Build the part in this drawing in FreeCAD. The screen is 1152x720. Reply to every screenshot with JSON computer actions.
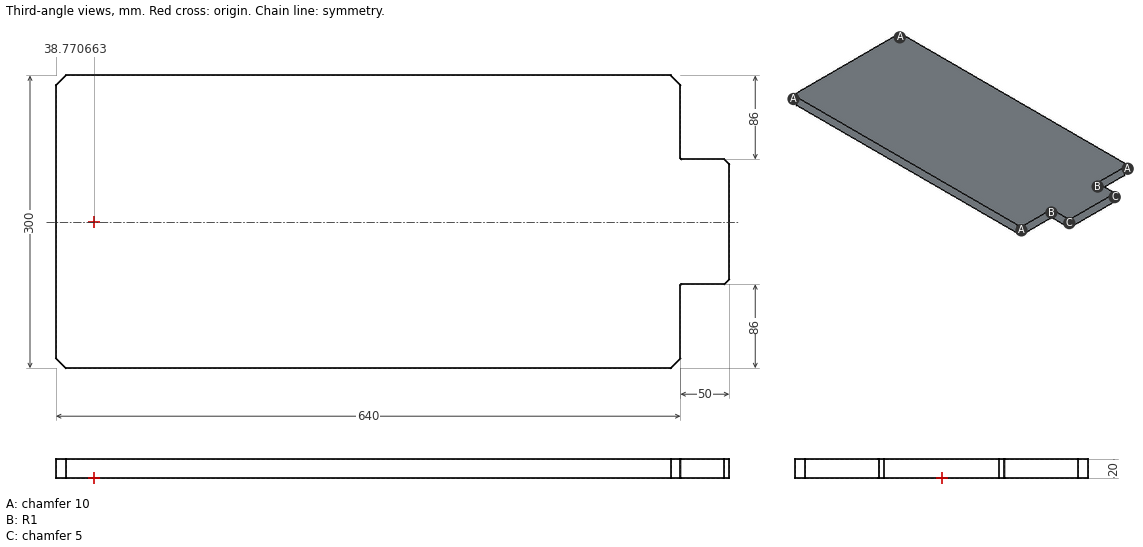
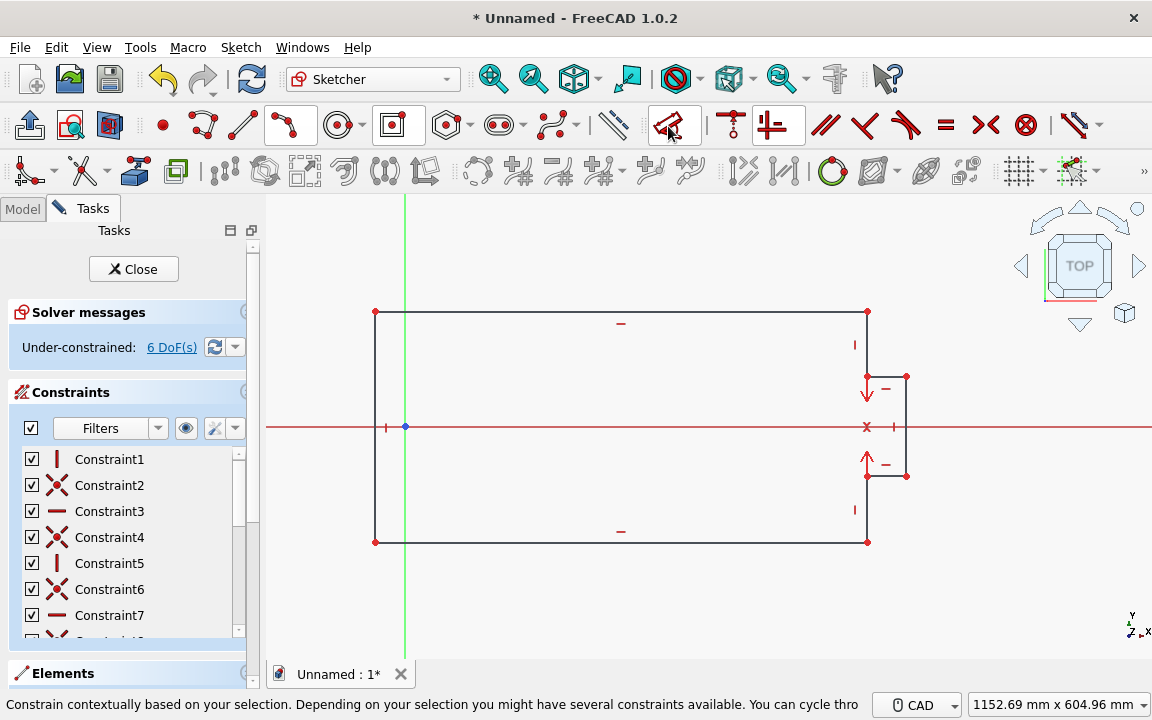
{"action": "left_click", "coordinate": [867, 523]}
{"action": "left_click", "coordinate": [901, 510]}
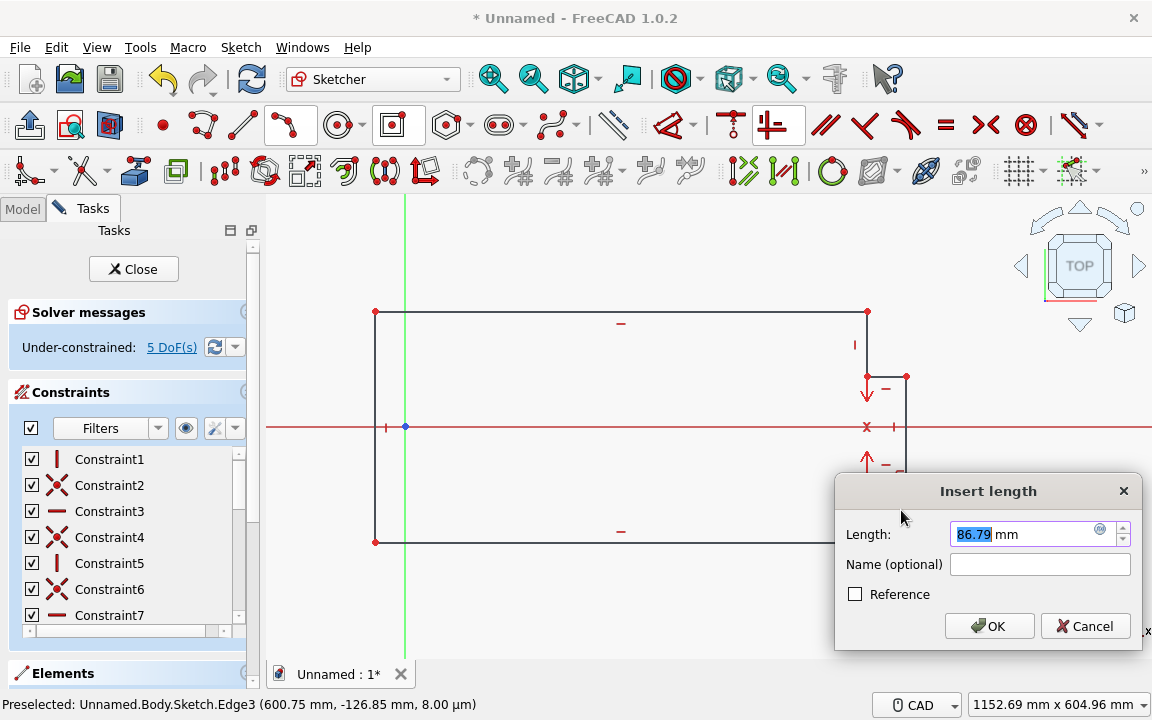
{"action": "type", "text": "86"}
{"action": "key", "text": "Return"}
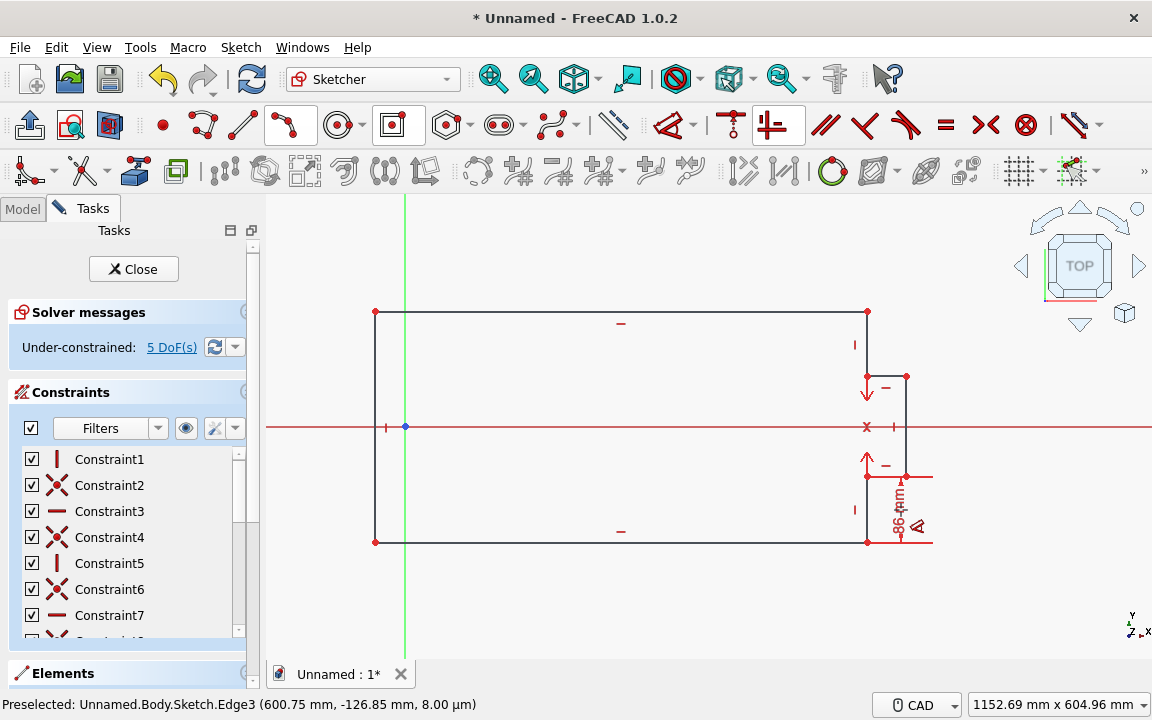
{"action": "left_click", "coordinate": [879, 477]}
{"action": "left_click", "coordinate": [886, 443]}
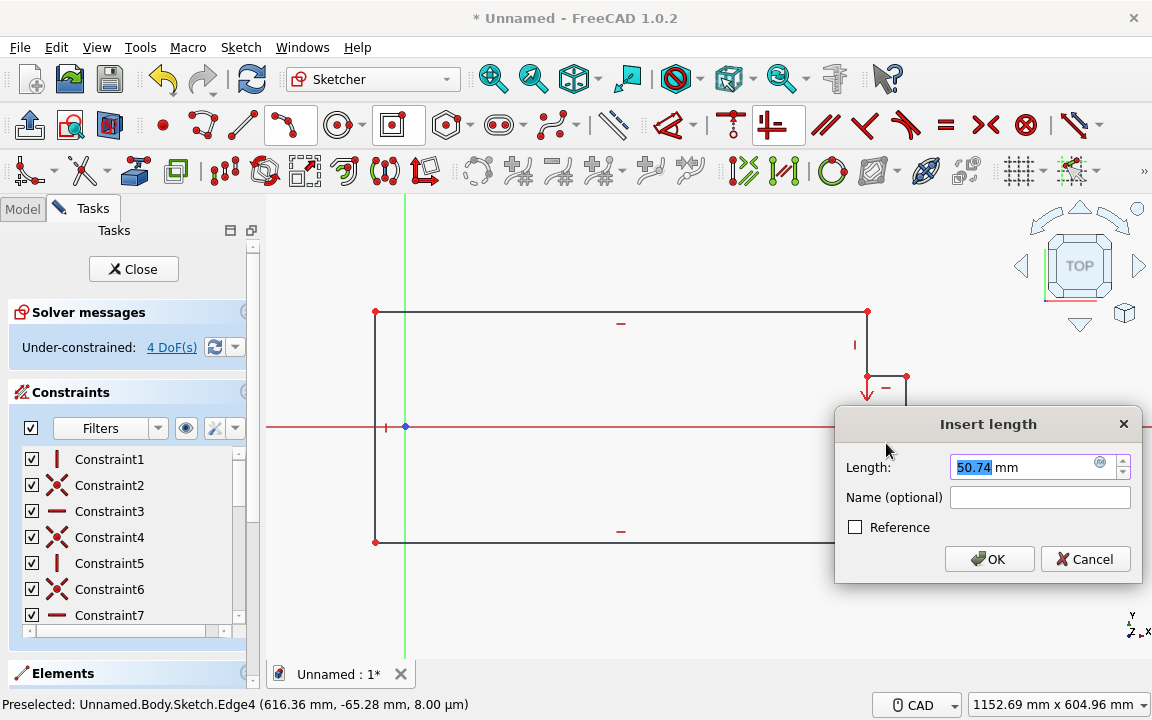
{"action": "type", "text": "50"}
{"action": "key", "text": "Return"}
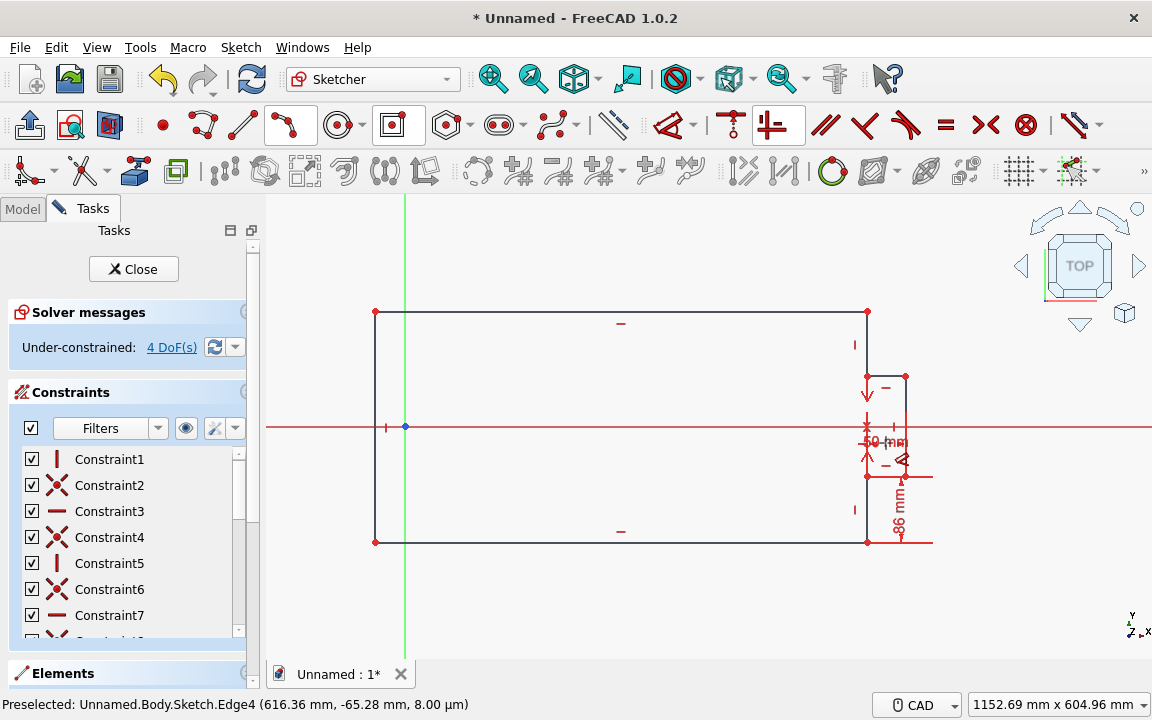
{"action": "left_click", "coordinate": [867, 357]}
{"action": "left_click", "coordinate": [901, 344]}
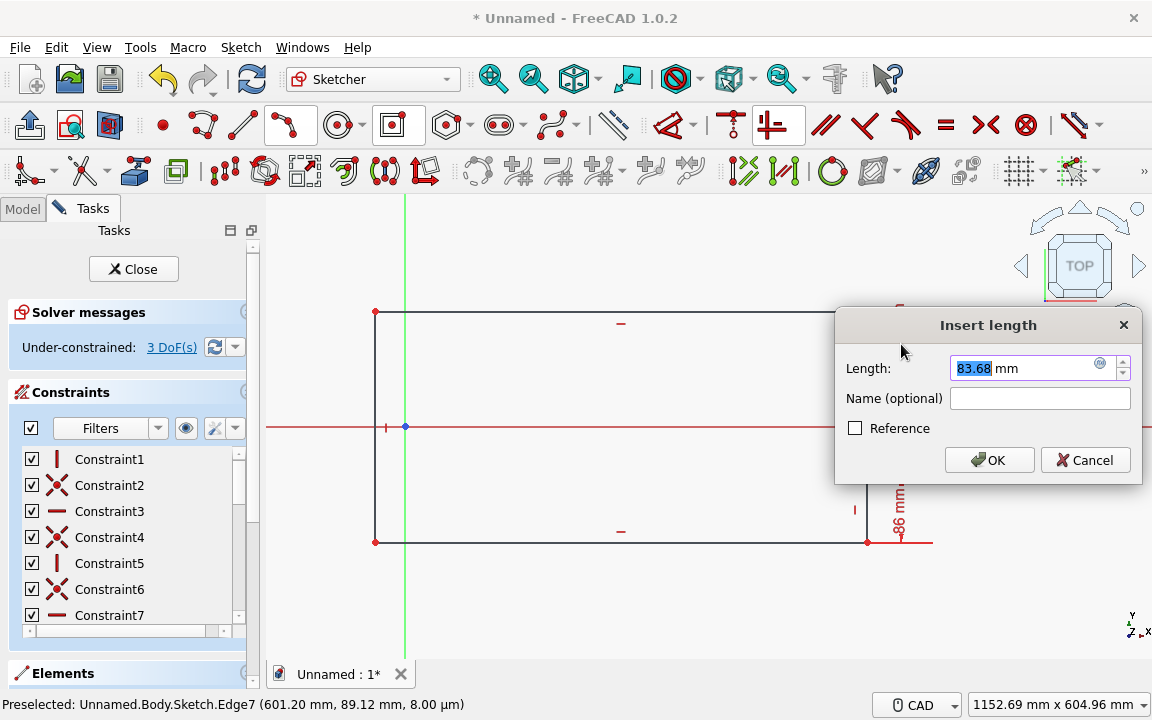
{"action": "type", "text": "86"}
{"action": "key", "text": "Return"}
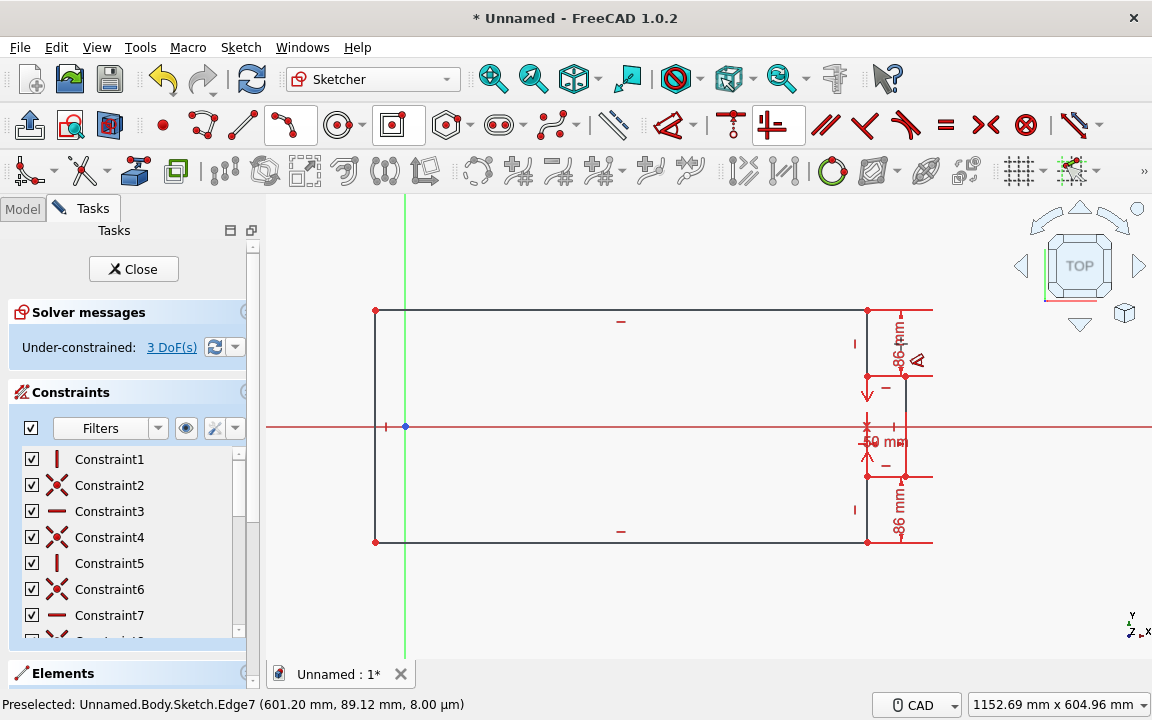
{"action": "left_click", "coordinate": [375, 380]}
{"action": "left_click", "coordinate": [341, 373]}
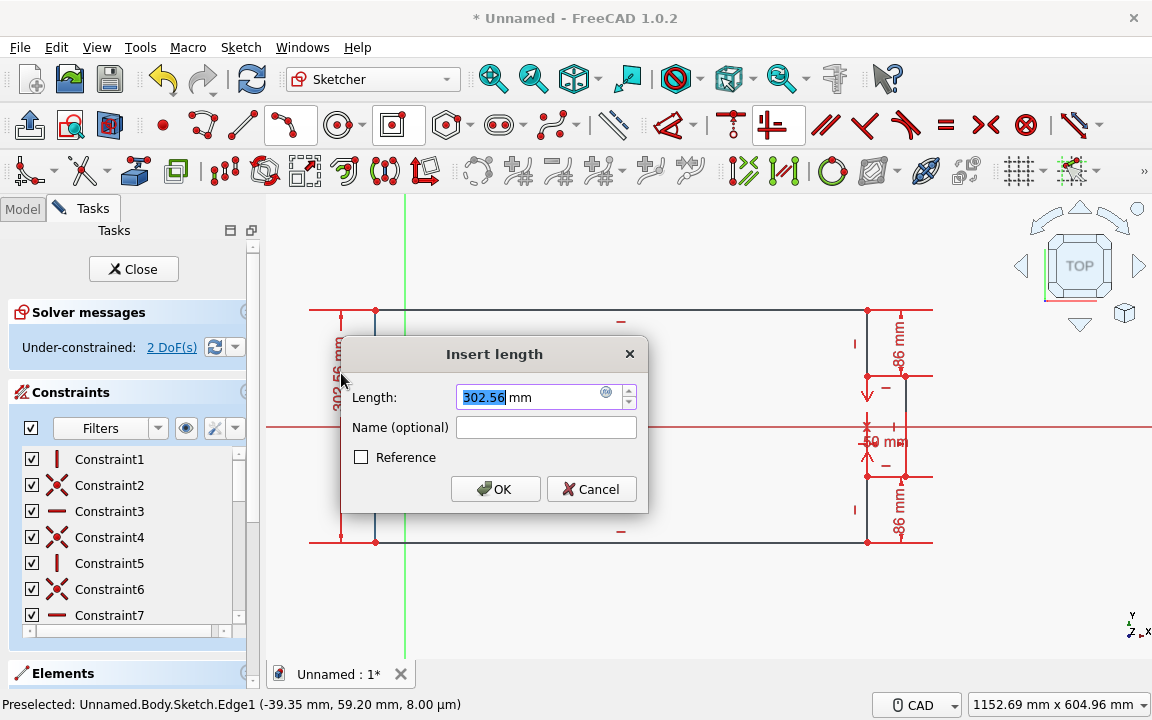
{"action": "type", "text": "300"}
{"action": "key", "text": "Return"}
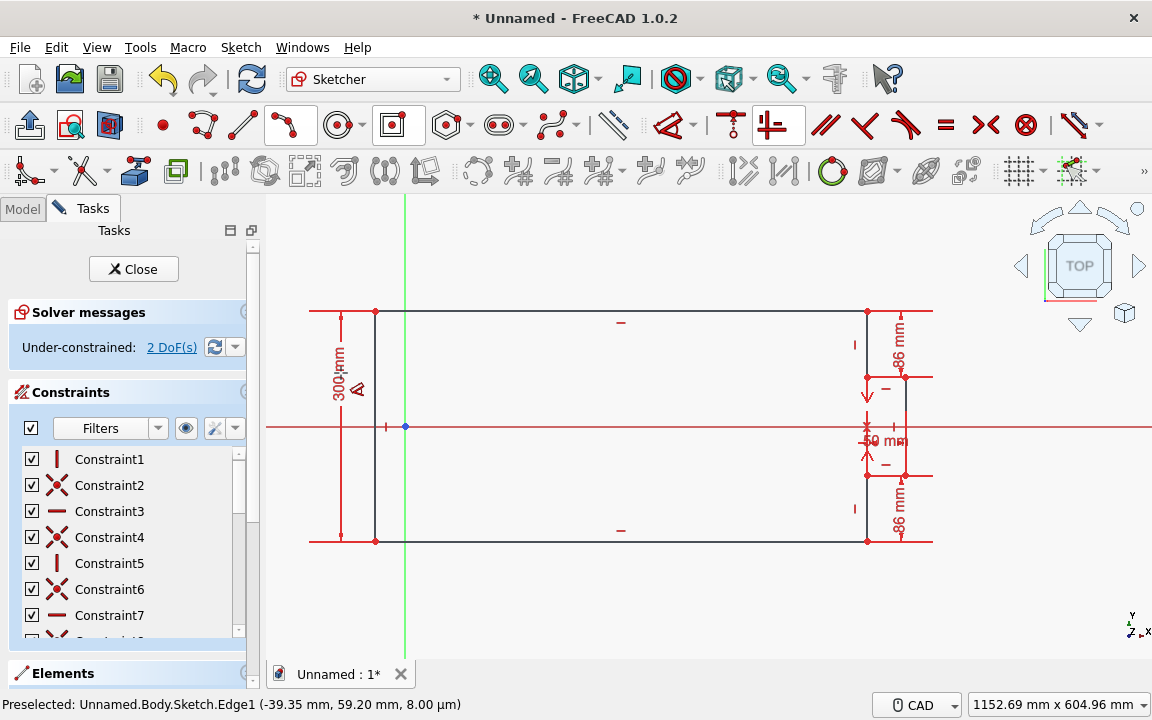
{"action": "left_click", "coordinate": [523, 542]}
{"action": "left_click", "coordinate": [621, 576]}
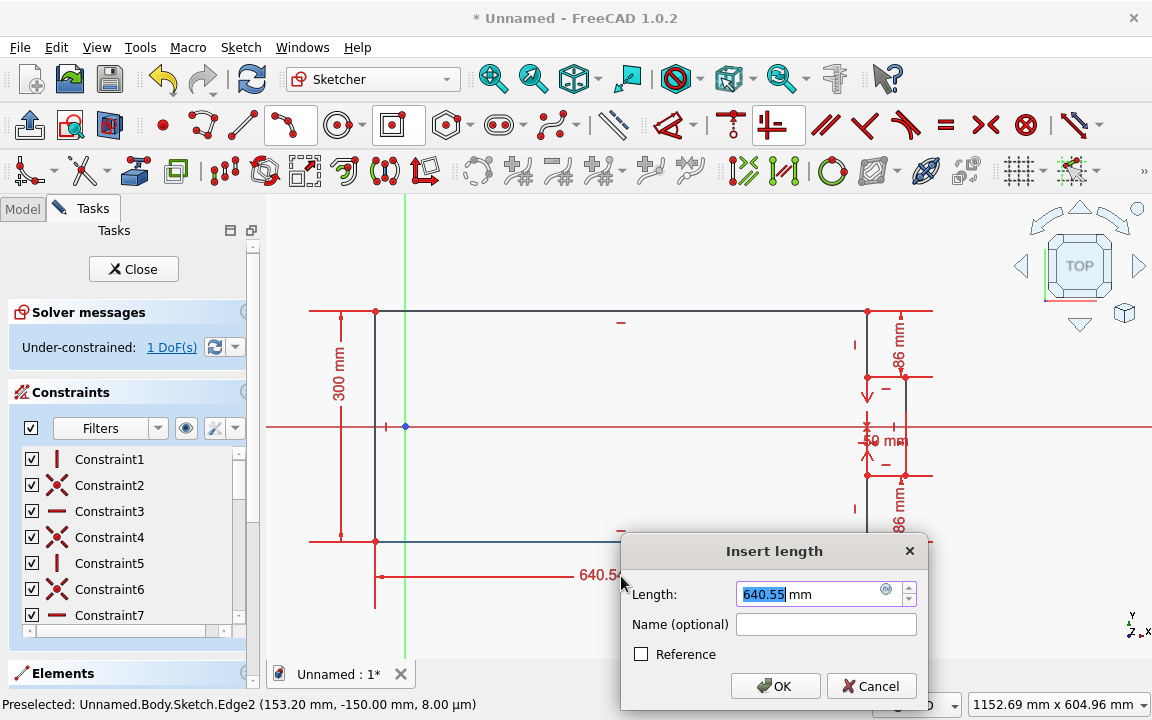
{"action": "type", "text": "640"}
{"action": "key", "text": "Return"}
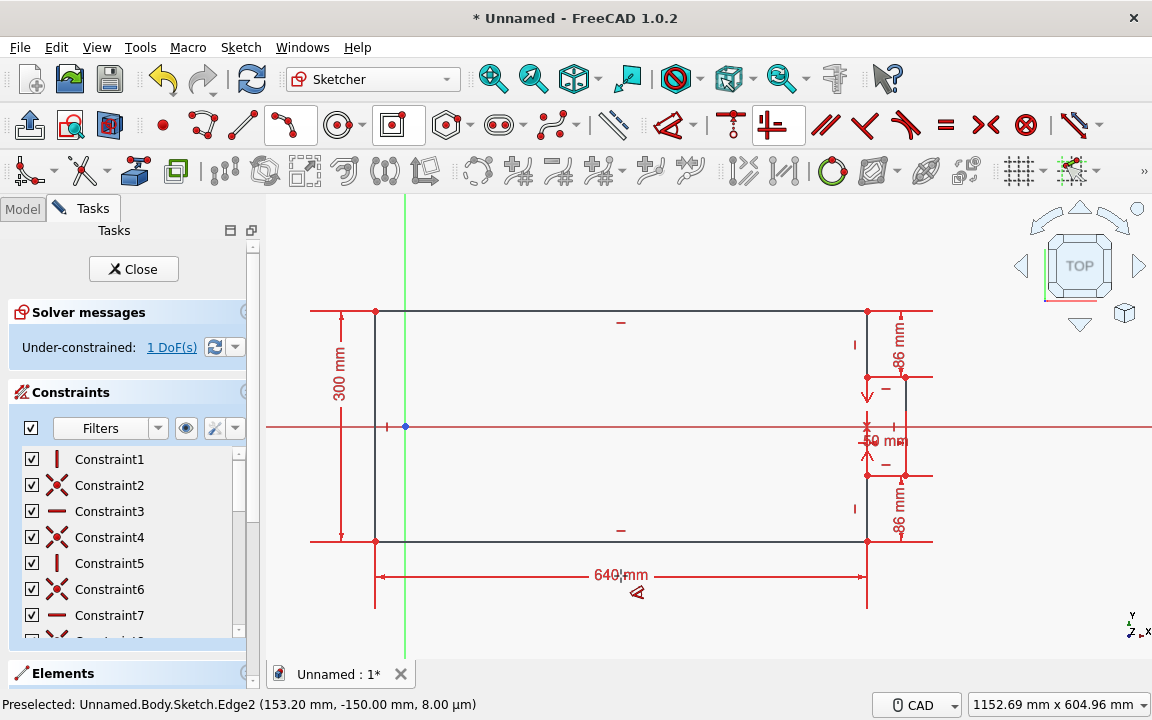
{"action": "scroll", "coordinate": [375, 311], "scroll_direction": "up", "scroll_amount": 2}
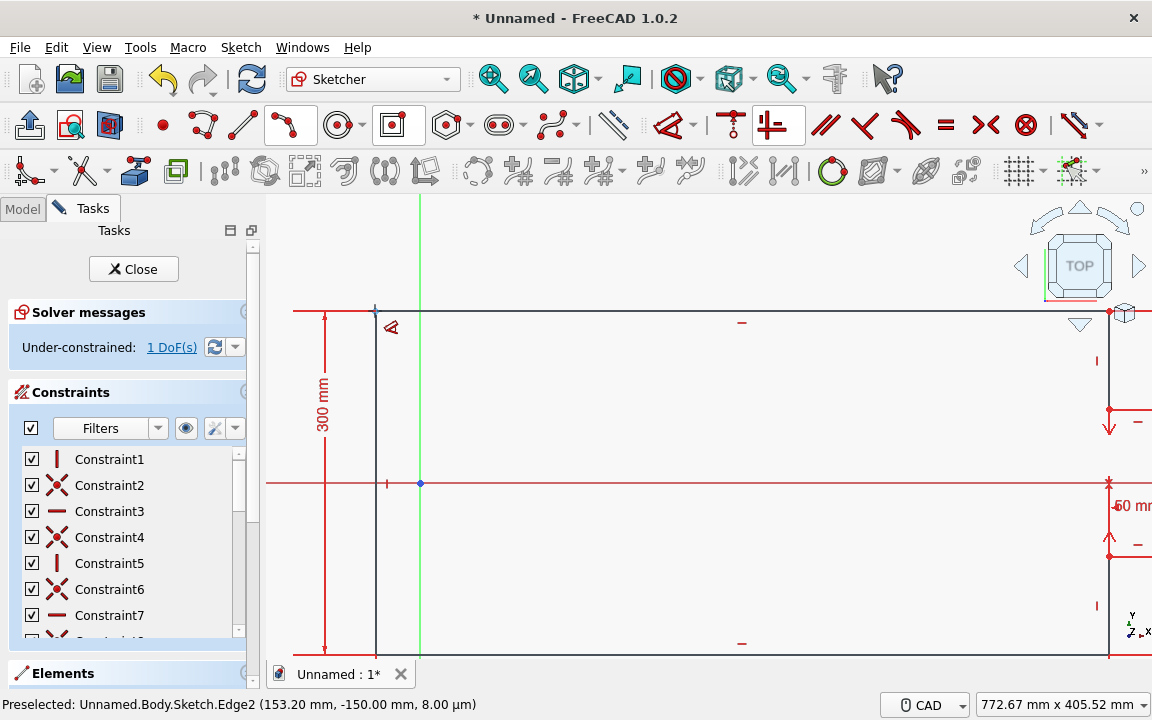
{"action": "left_click", "coordinate": [376, 311]}
{"action": "left_click", "coordinate": [398, 277]}